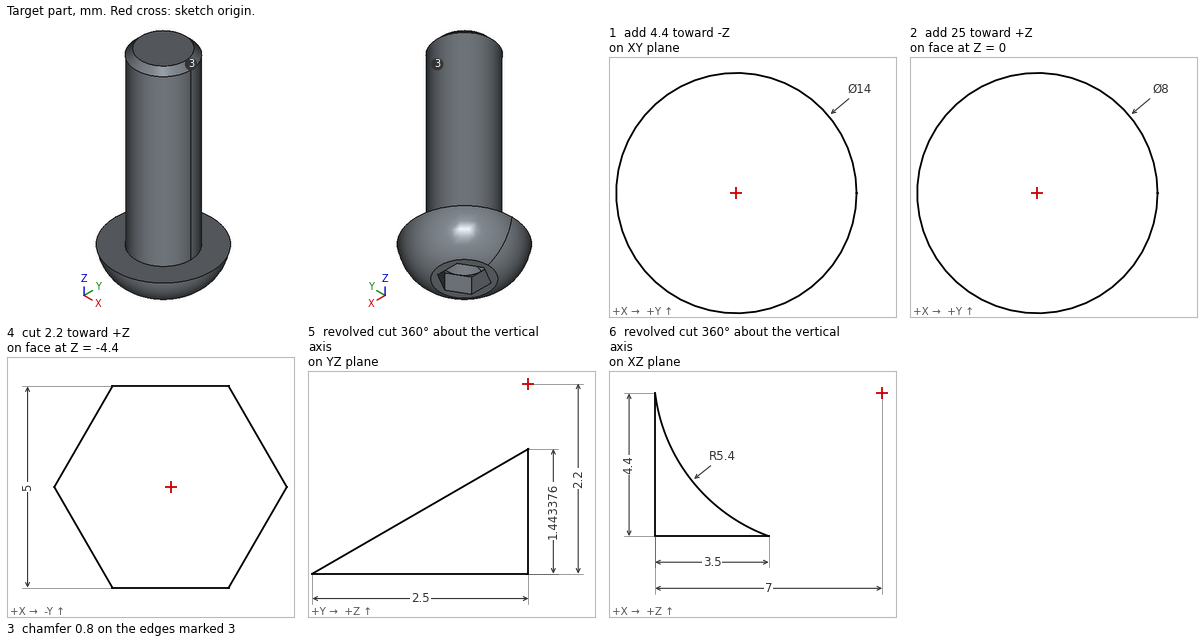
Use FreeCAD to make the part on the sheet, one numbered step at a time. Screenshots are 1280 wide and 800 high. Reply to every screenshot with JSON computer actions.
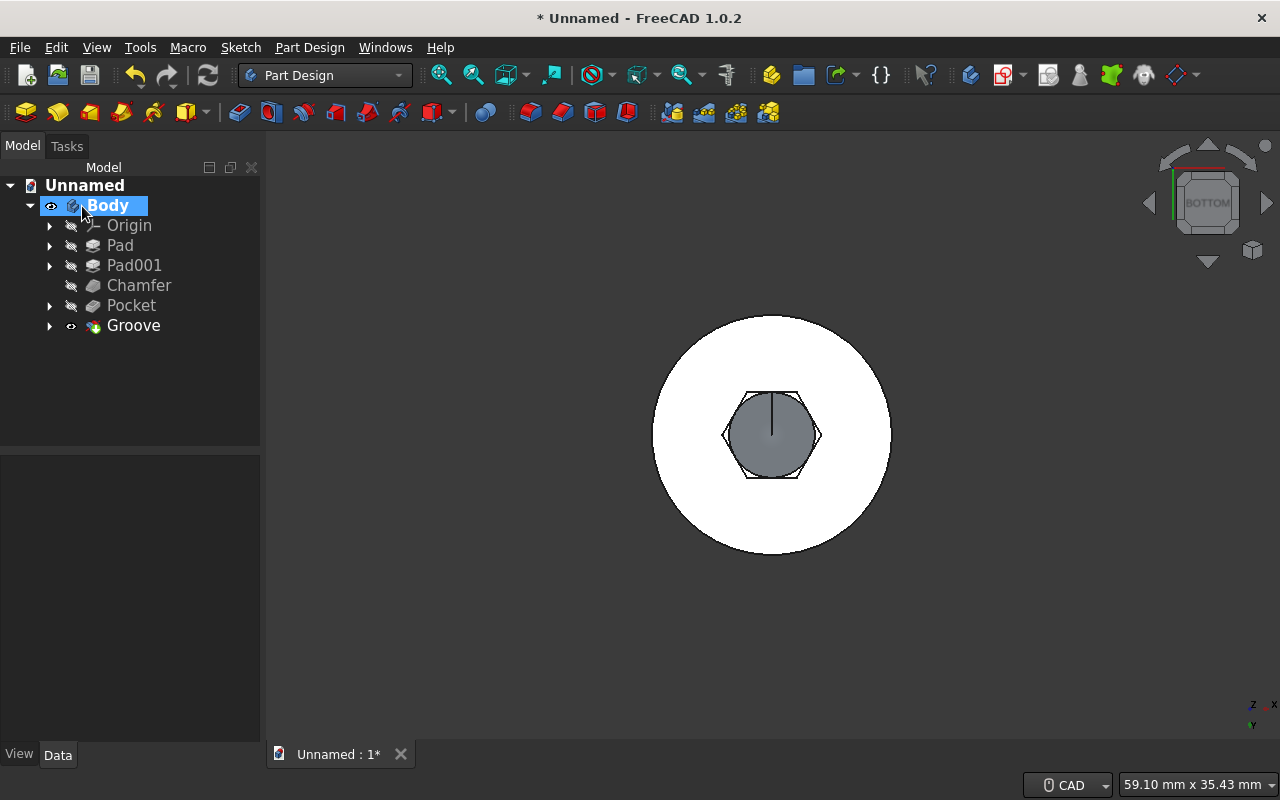
{"action": "left_click", "coordinate": [442, 76]}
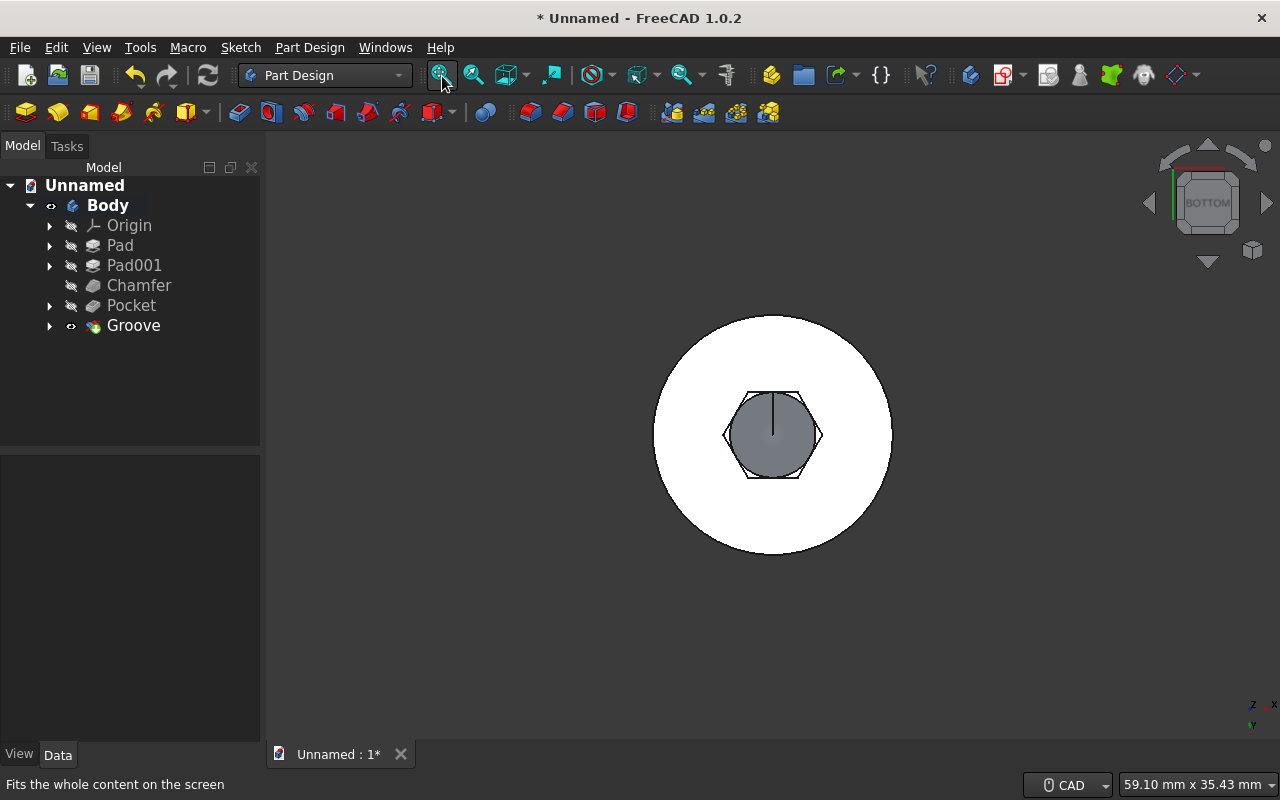
{"action": "left_click", "coordinate": [1004, 76]}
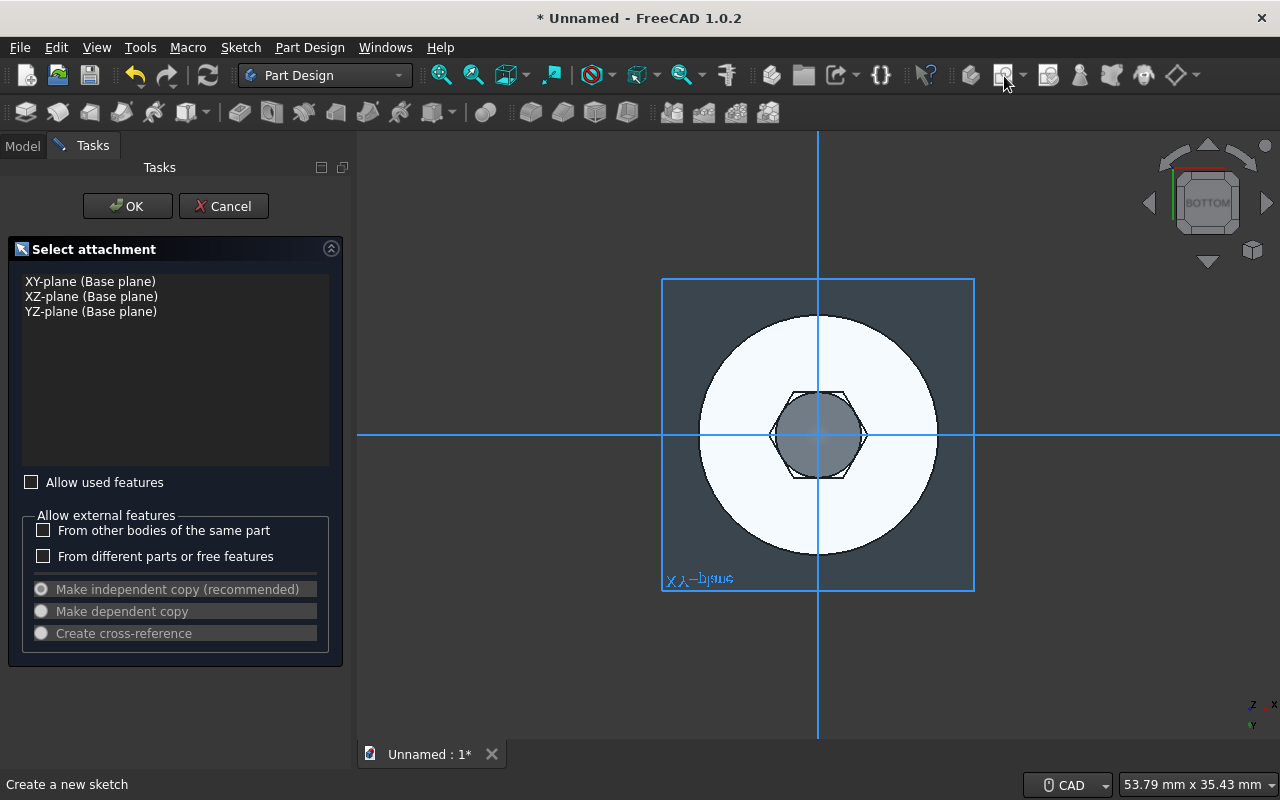
{"action": "left_click", "coordinate": [82, 296]}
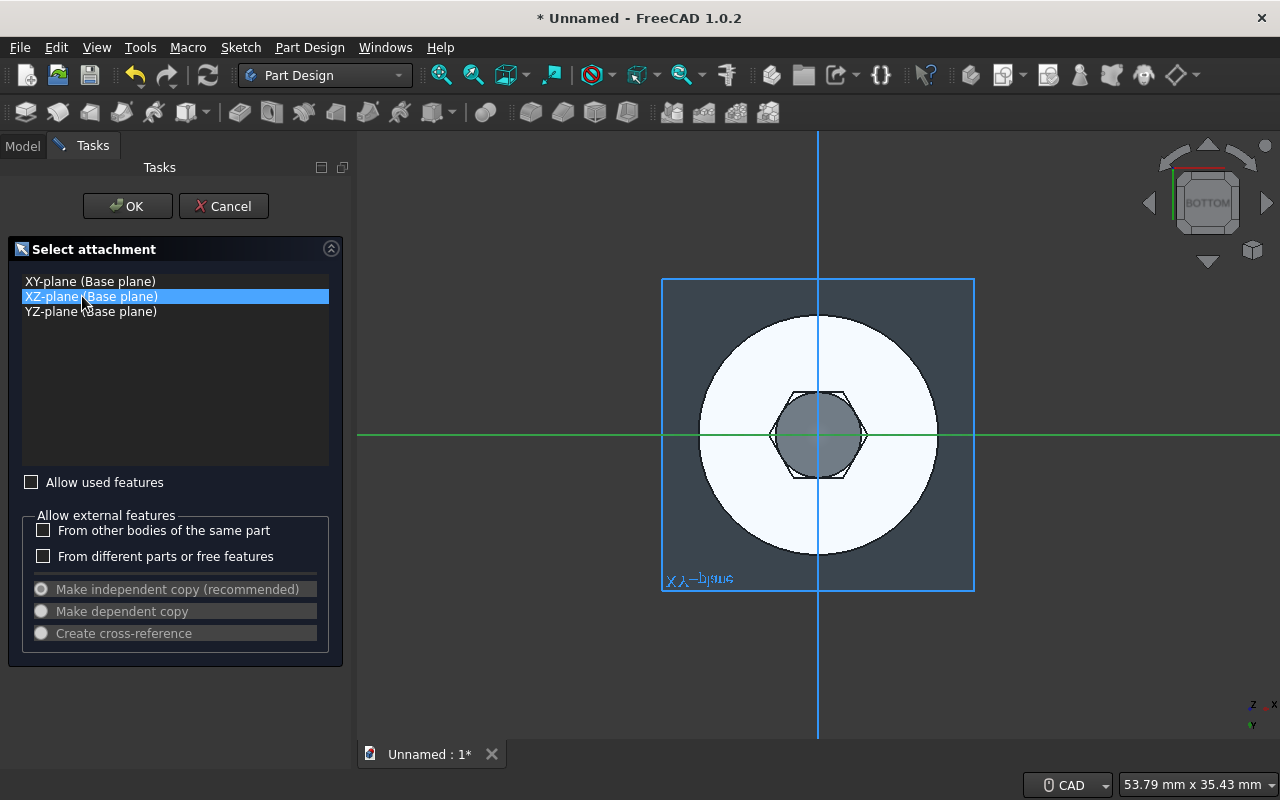
{"action": "left_click", "coordinate": [128, 206]}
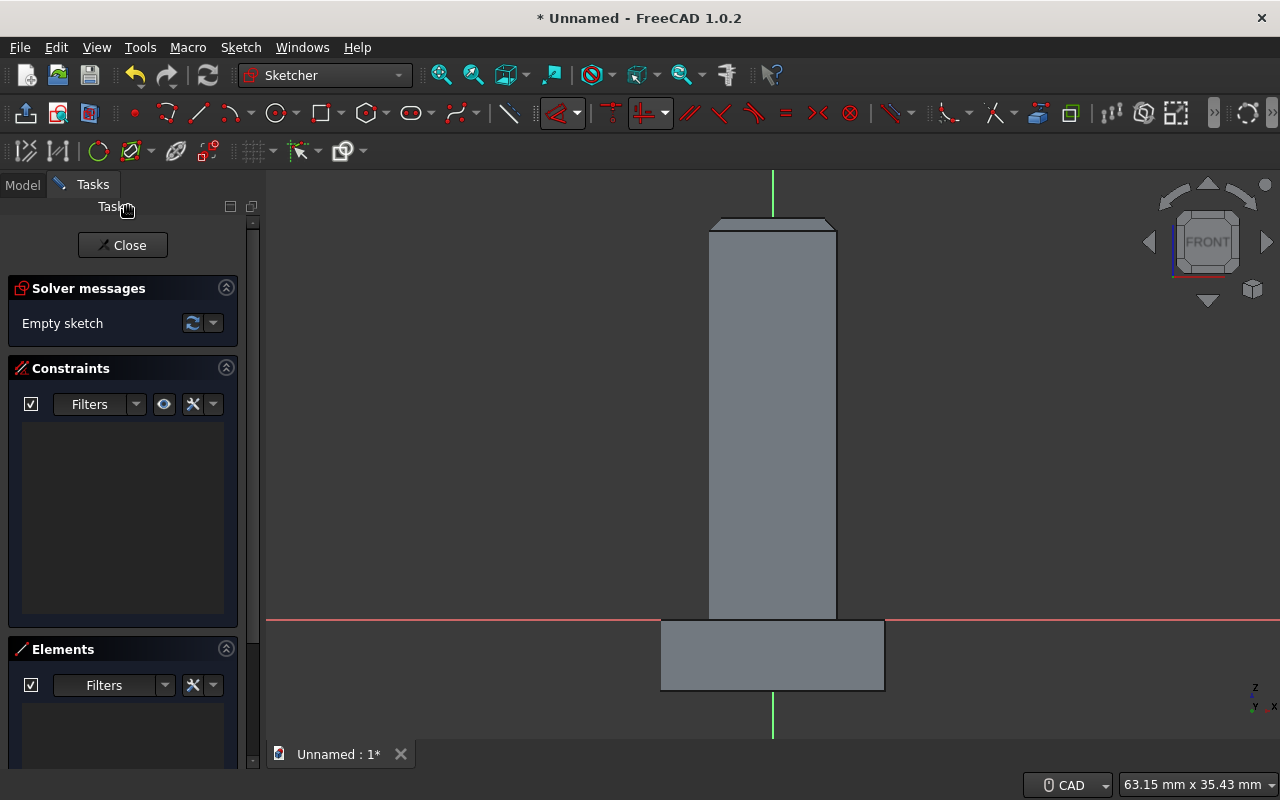
{"action": "key", "text": "q s"}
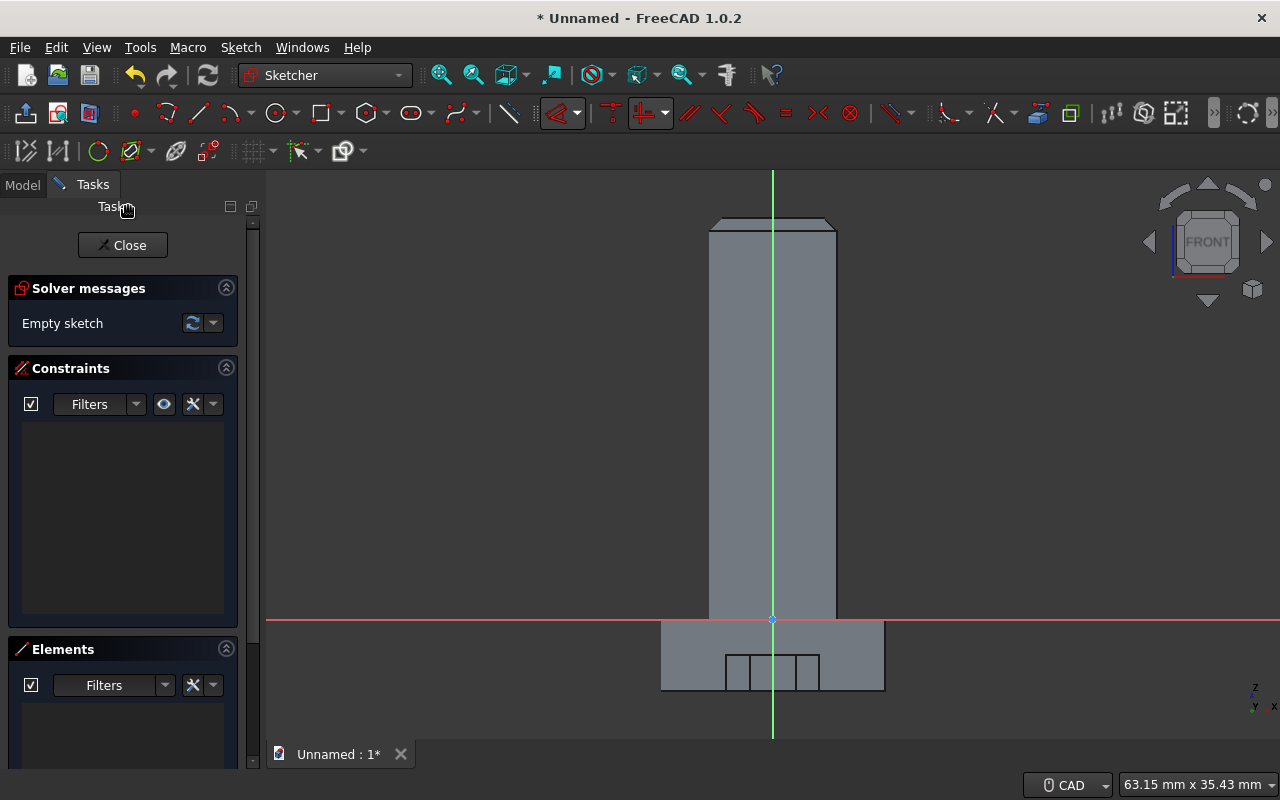
{"action": "scroll", "coordinate": [720, 706], "scroll_direction": "up", "scroll_amount": 8}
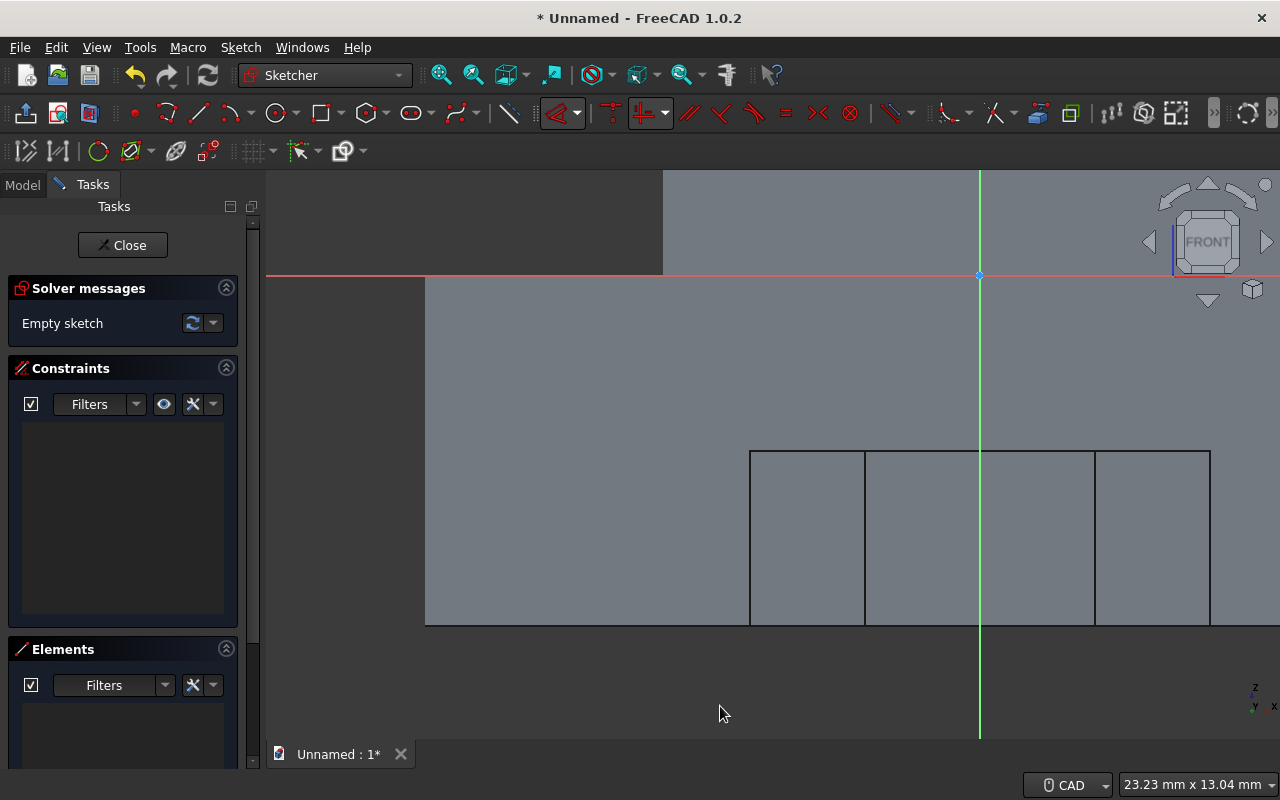
{"action": "left_click", "coordinate": [168, 114]}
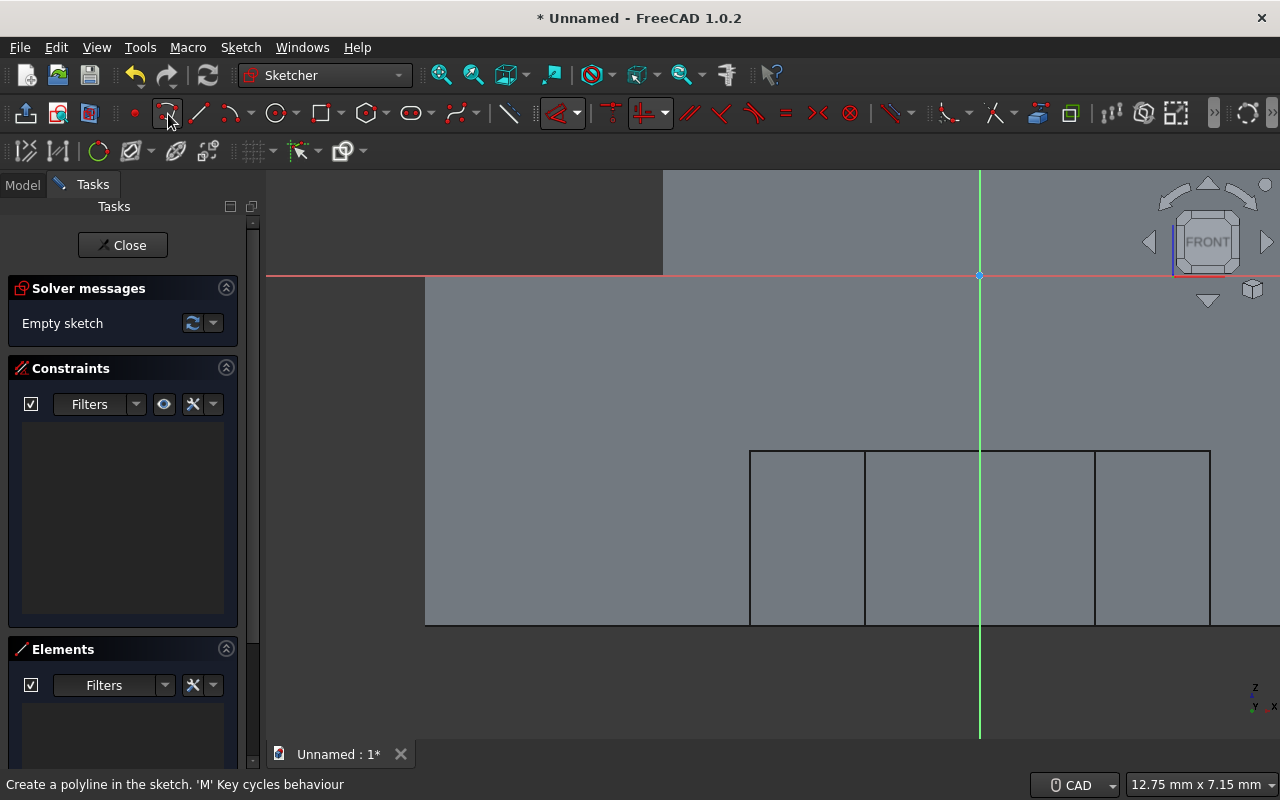
{"action": "left_click", "coordinate": [702, 626]}
{"action": "left_click", "coordinate": [423, 626]}
{"action": "left_click", "coordinate": [423, 276]}
{"action": "right_click", "coordinate": [423, 276]}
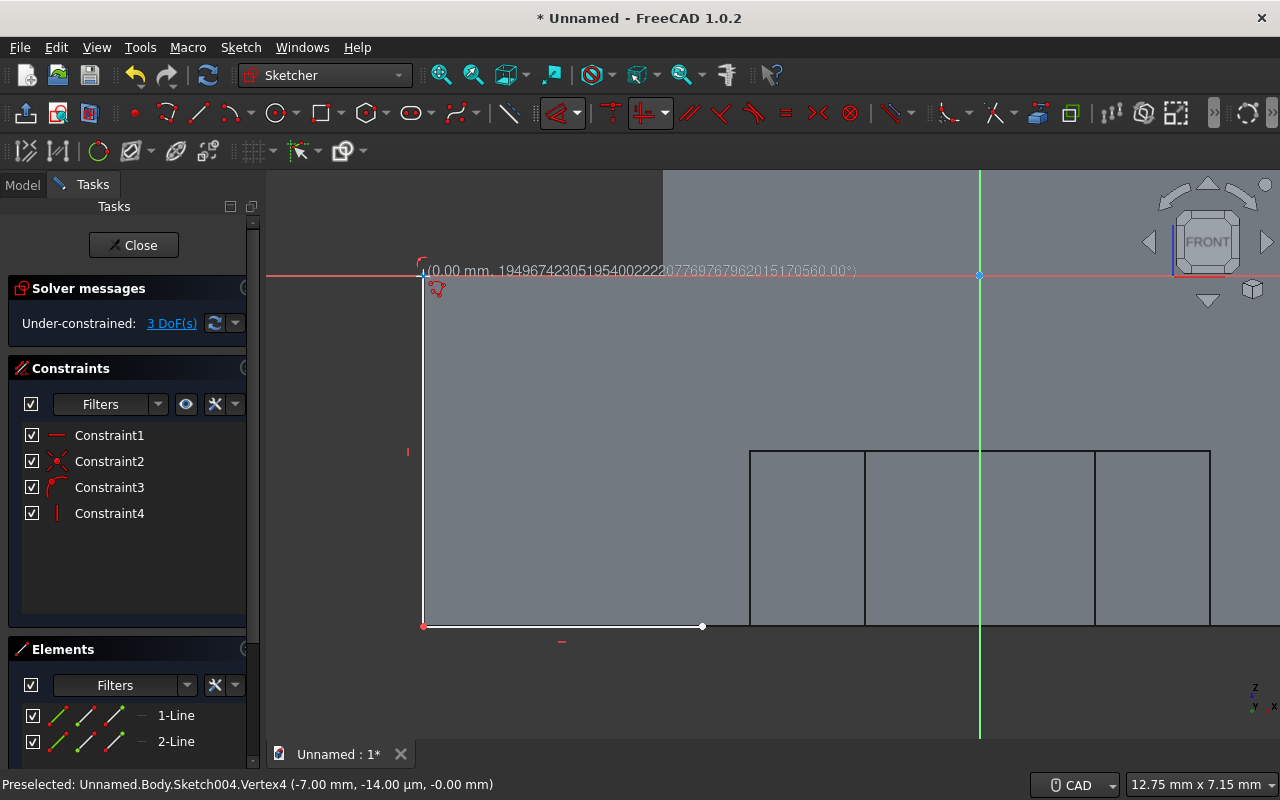
{"action": "left_click", "coordinate": [254, 114]}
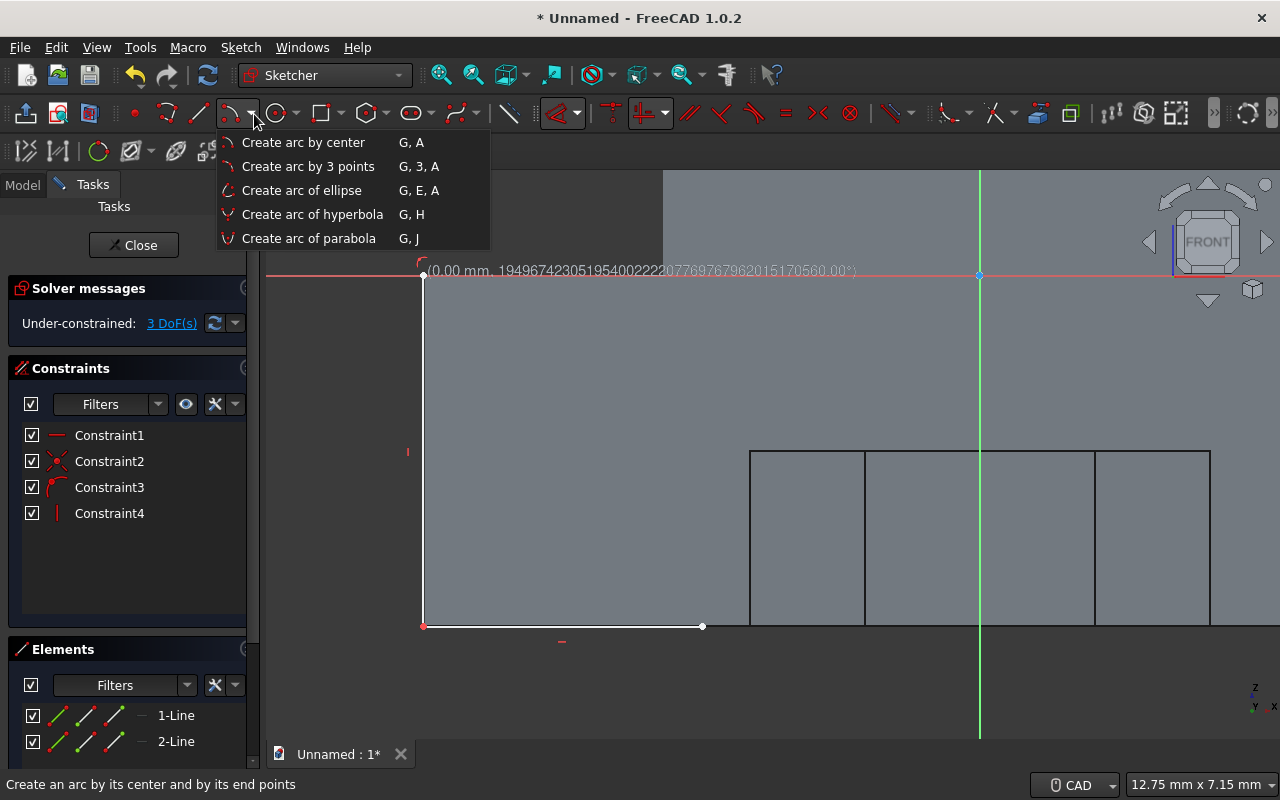
{"action": "left_click", "coordinate": [354, 166]}